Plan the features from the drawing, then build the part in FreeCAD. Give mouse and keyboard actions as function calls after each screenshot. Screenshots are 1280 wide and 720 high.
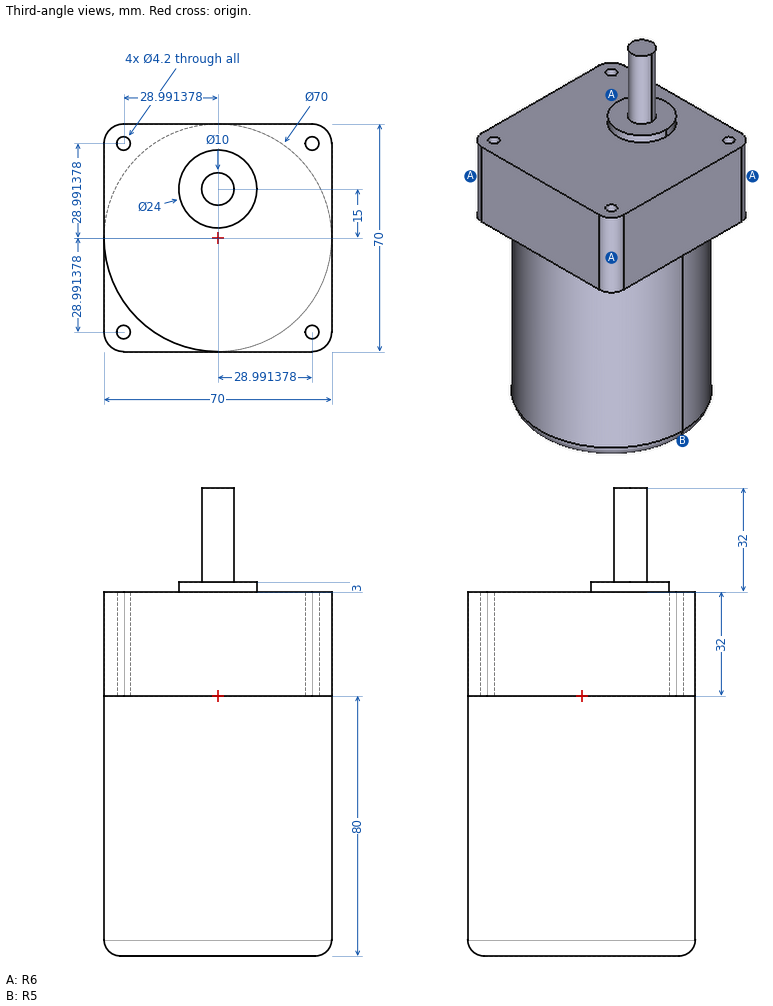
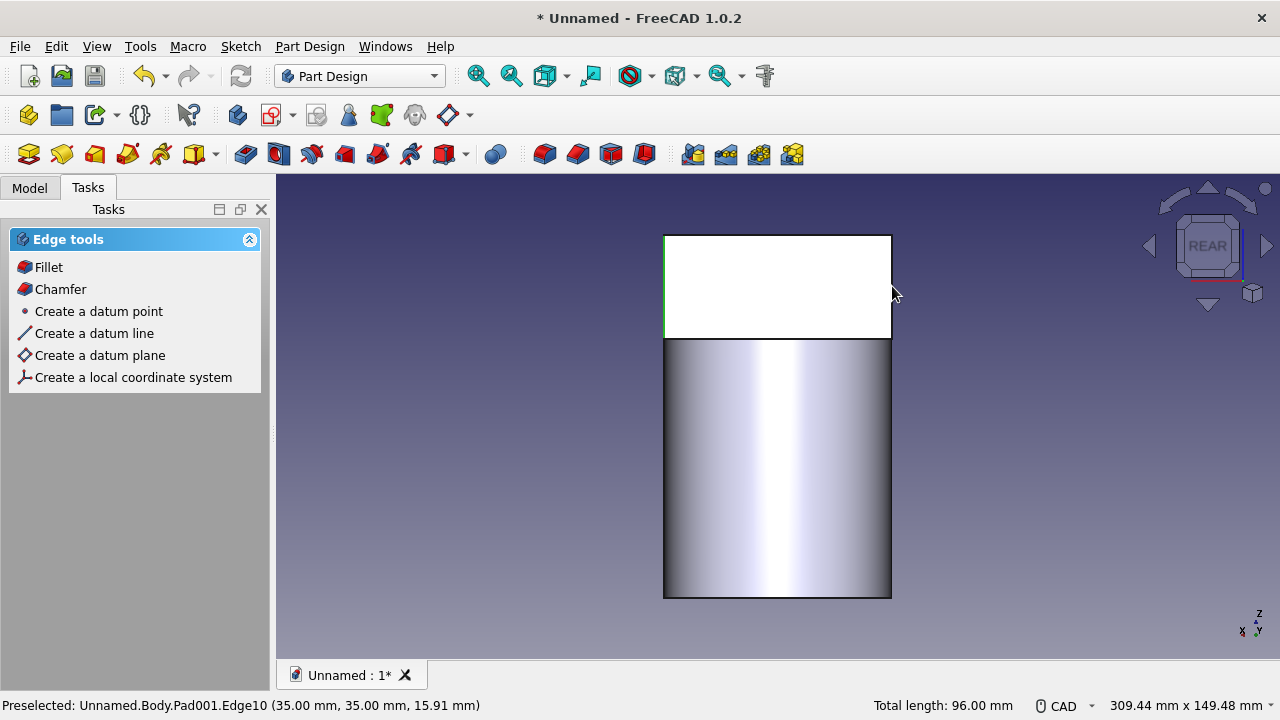
click(892, 286, ctrl)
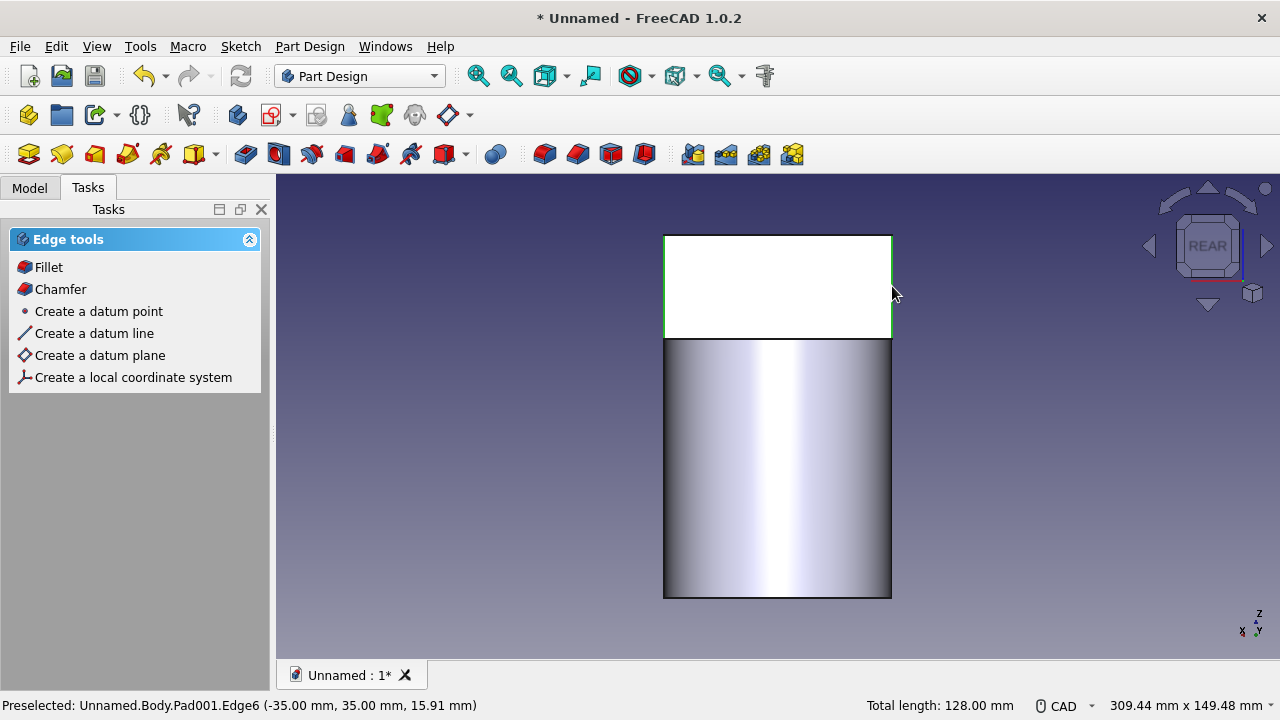
click(545, 154)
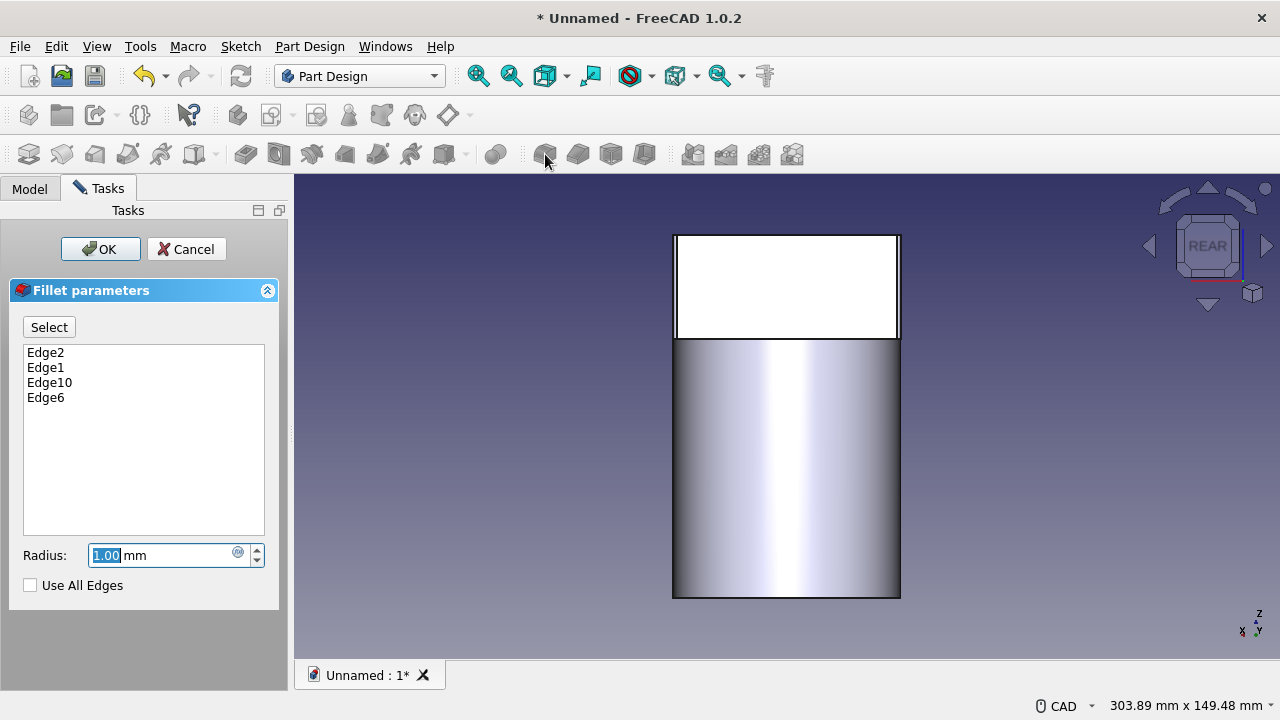
text(6)
key(Tab)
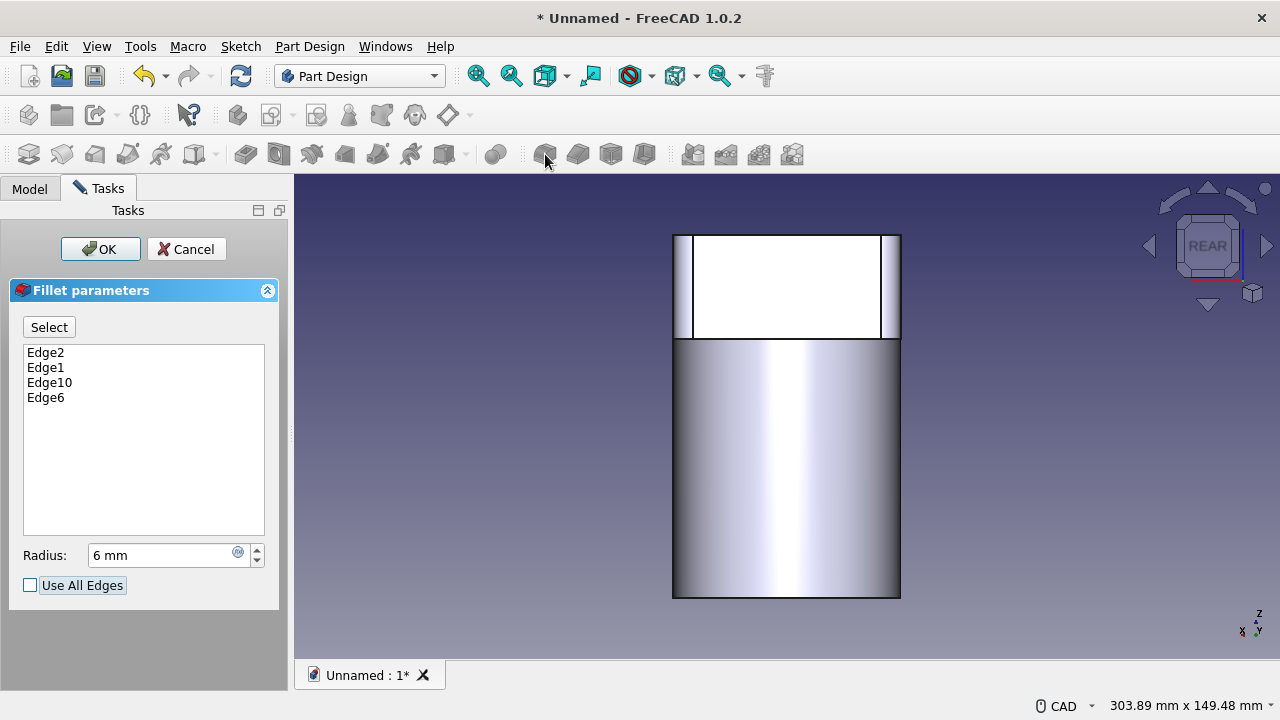
click(101, 249)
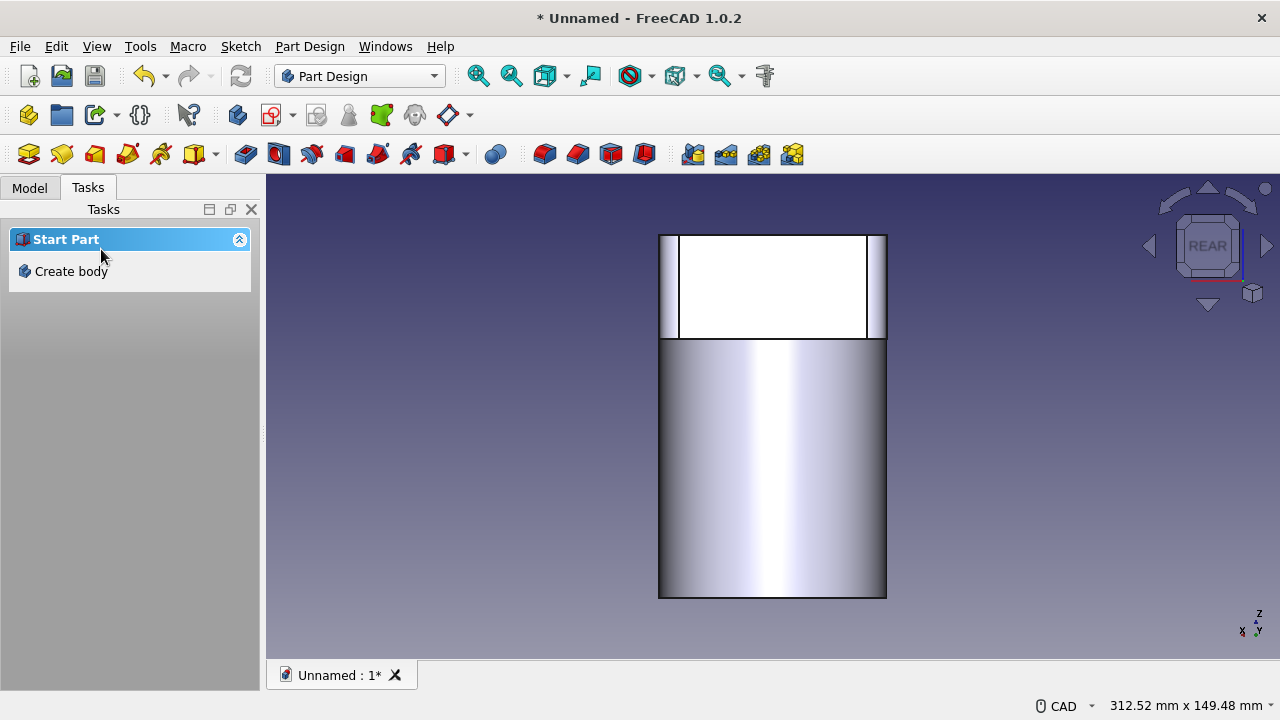
key(0)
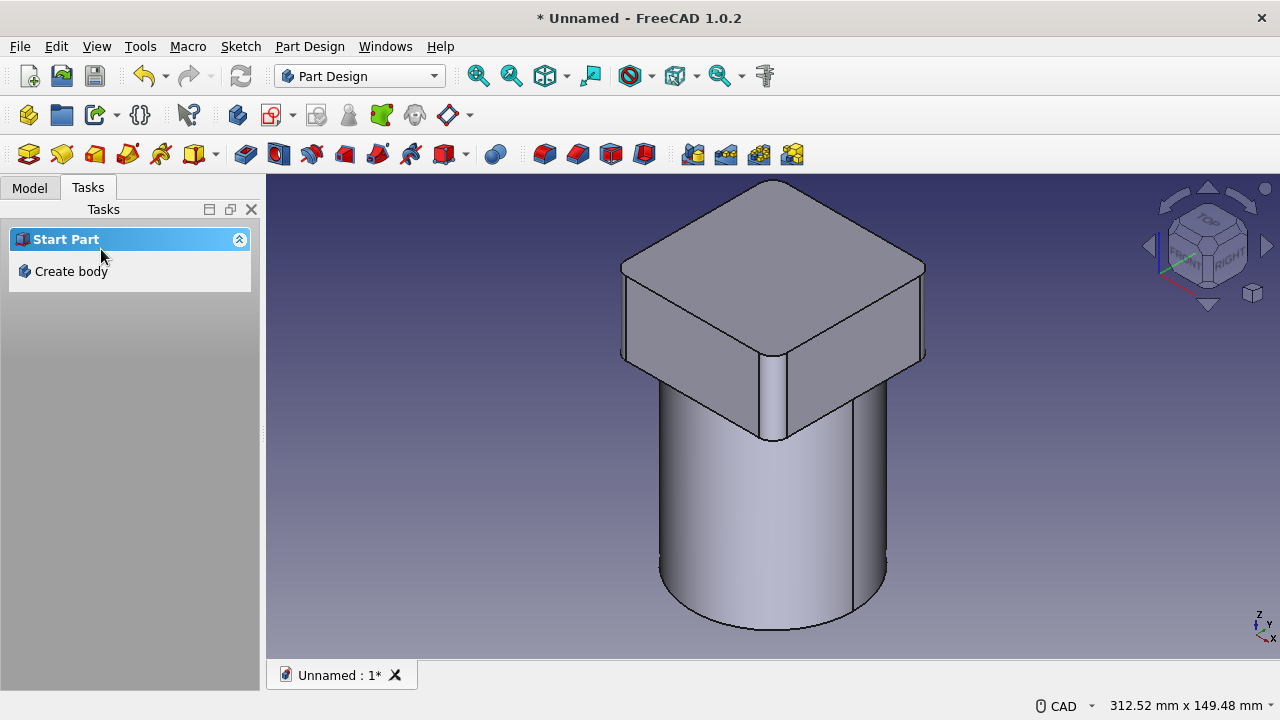
click(721, 622)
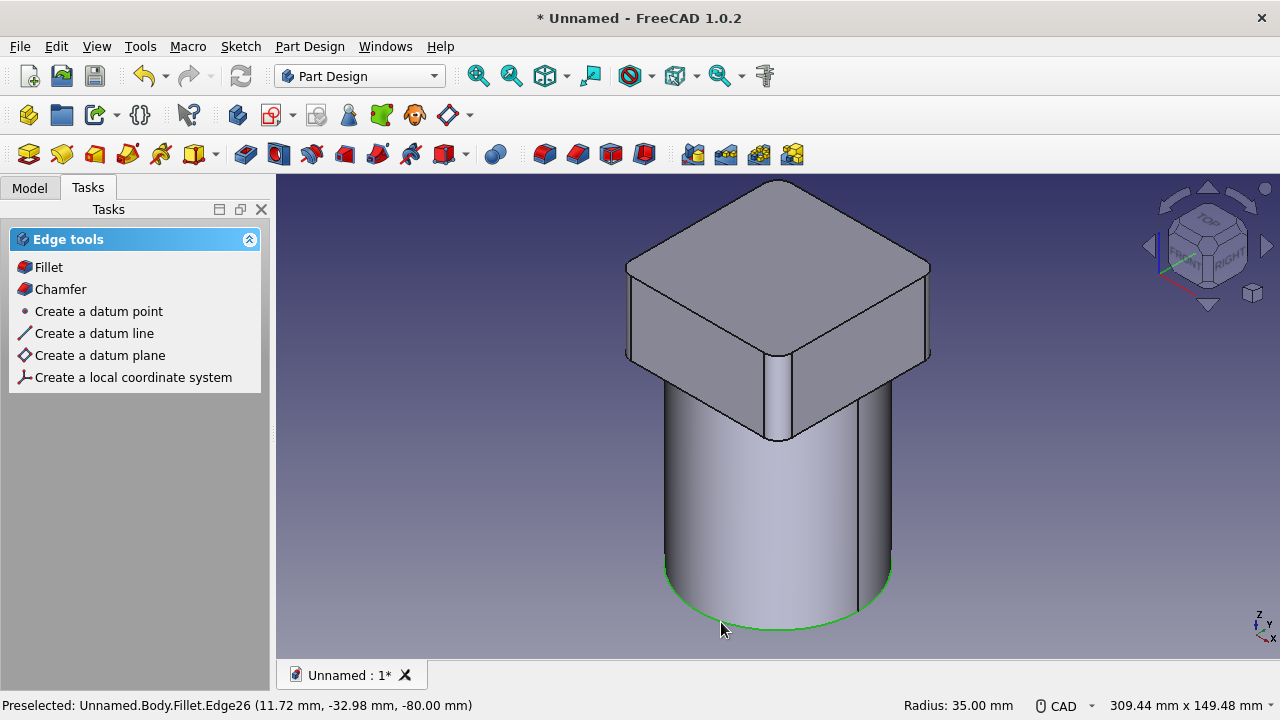
click(545, 154)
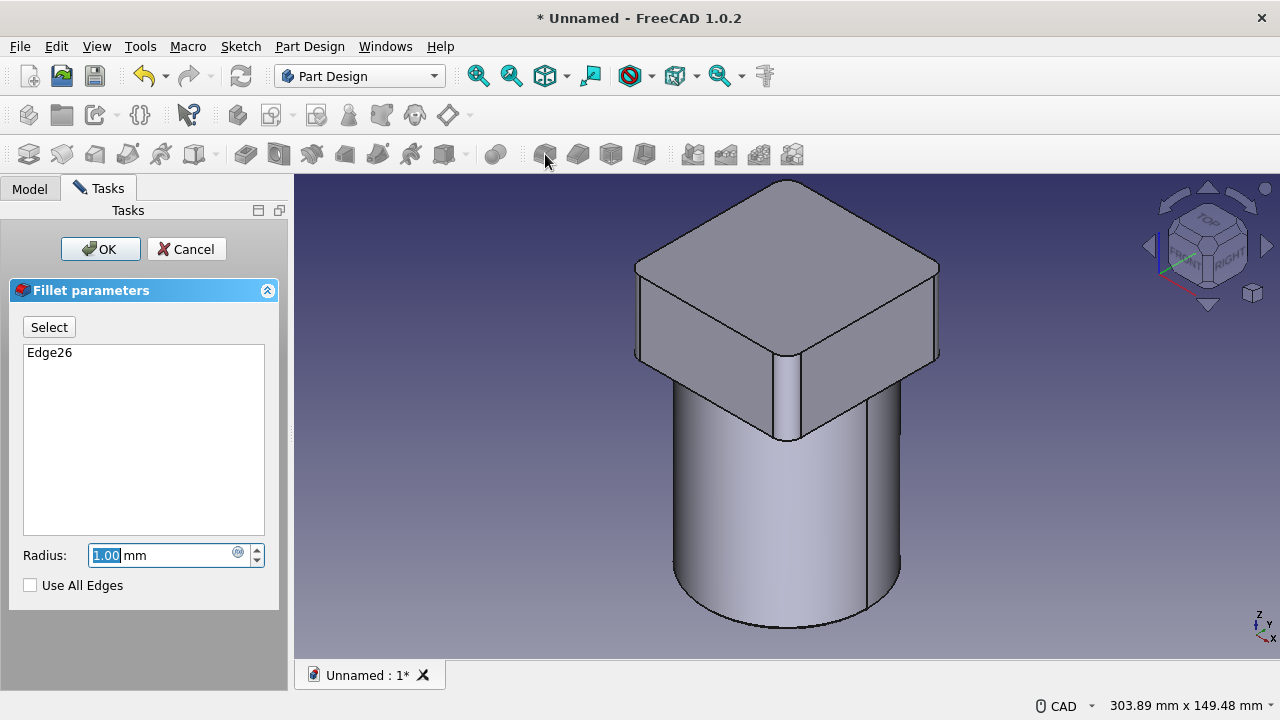
text(5)
key(Tab)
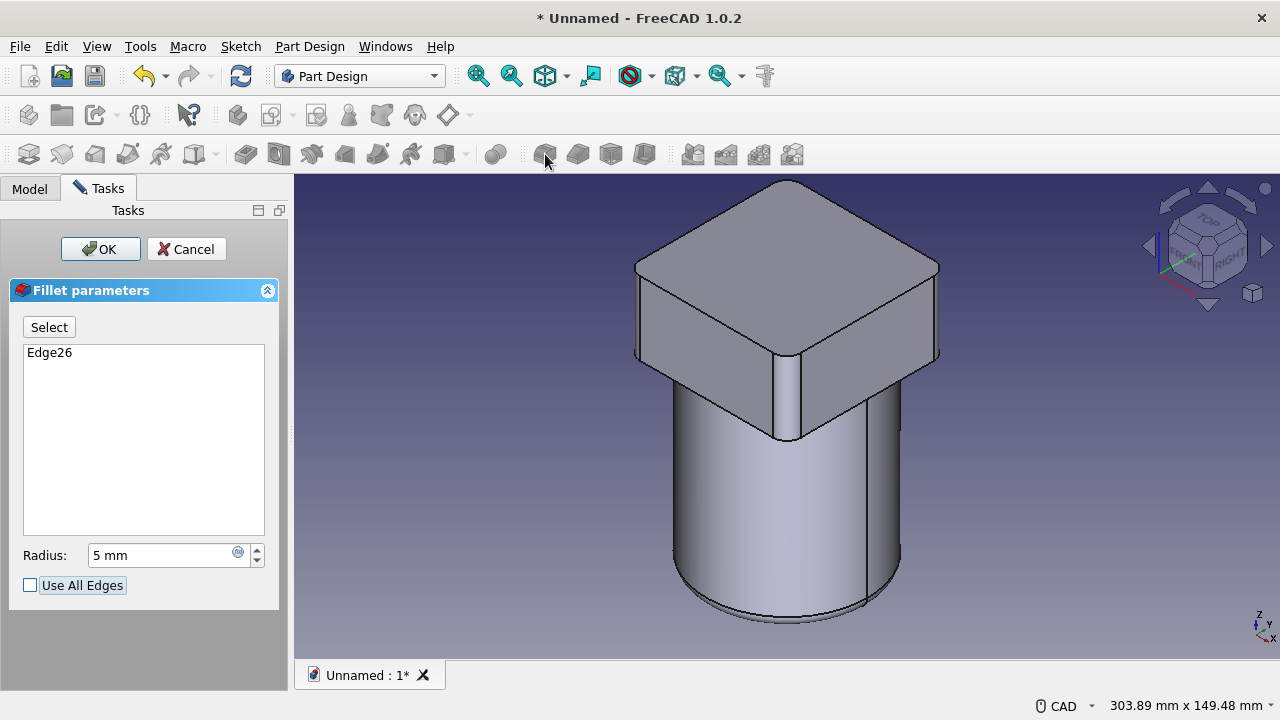
click(101, 249)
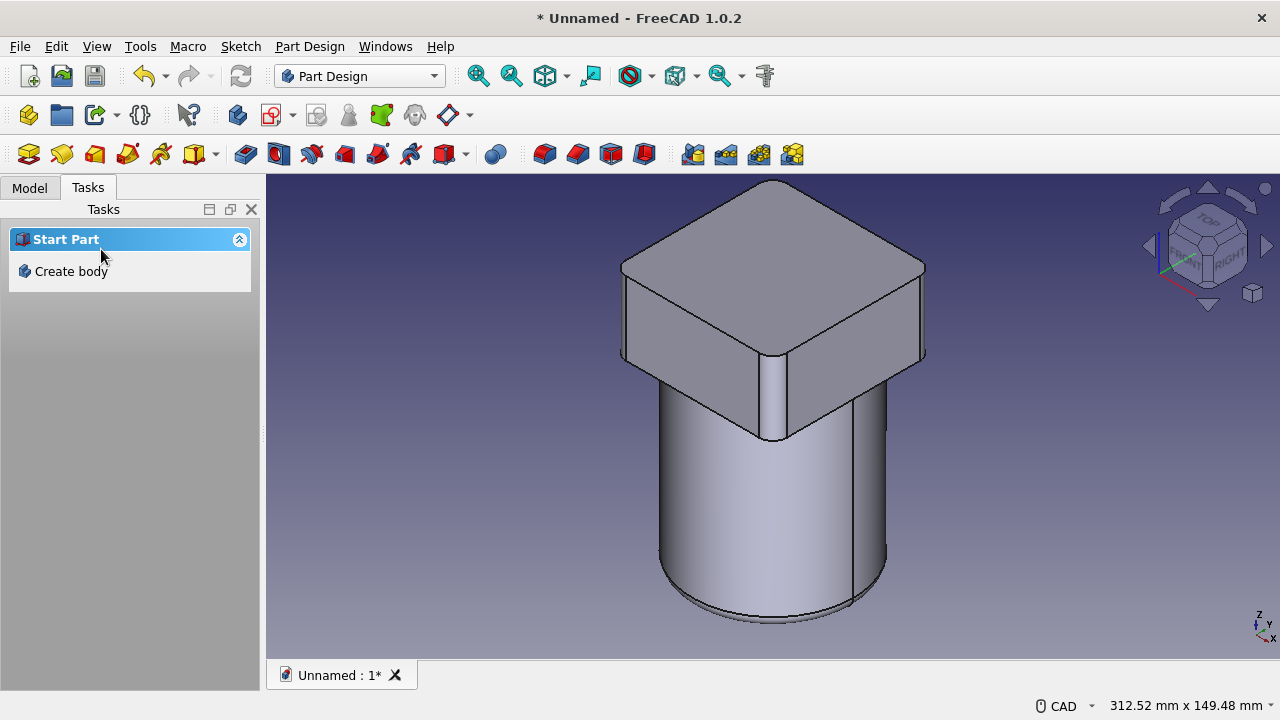
click(773, 267)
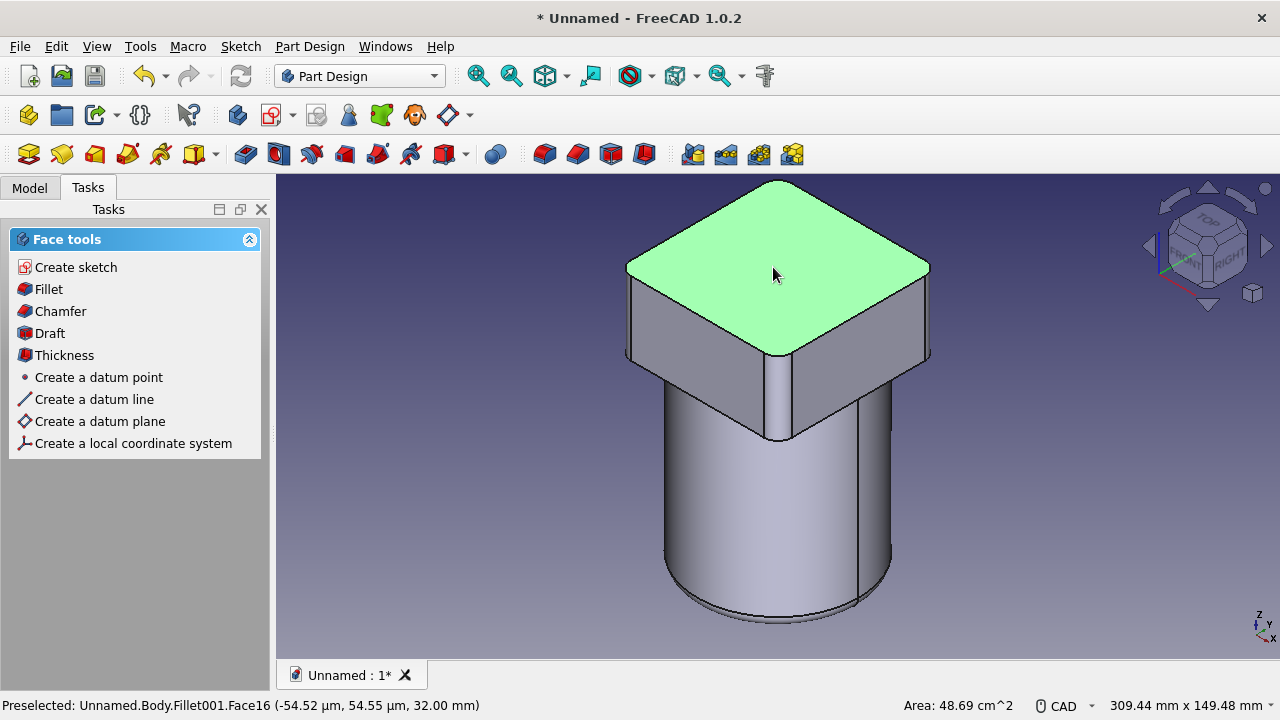
click(270, 116)